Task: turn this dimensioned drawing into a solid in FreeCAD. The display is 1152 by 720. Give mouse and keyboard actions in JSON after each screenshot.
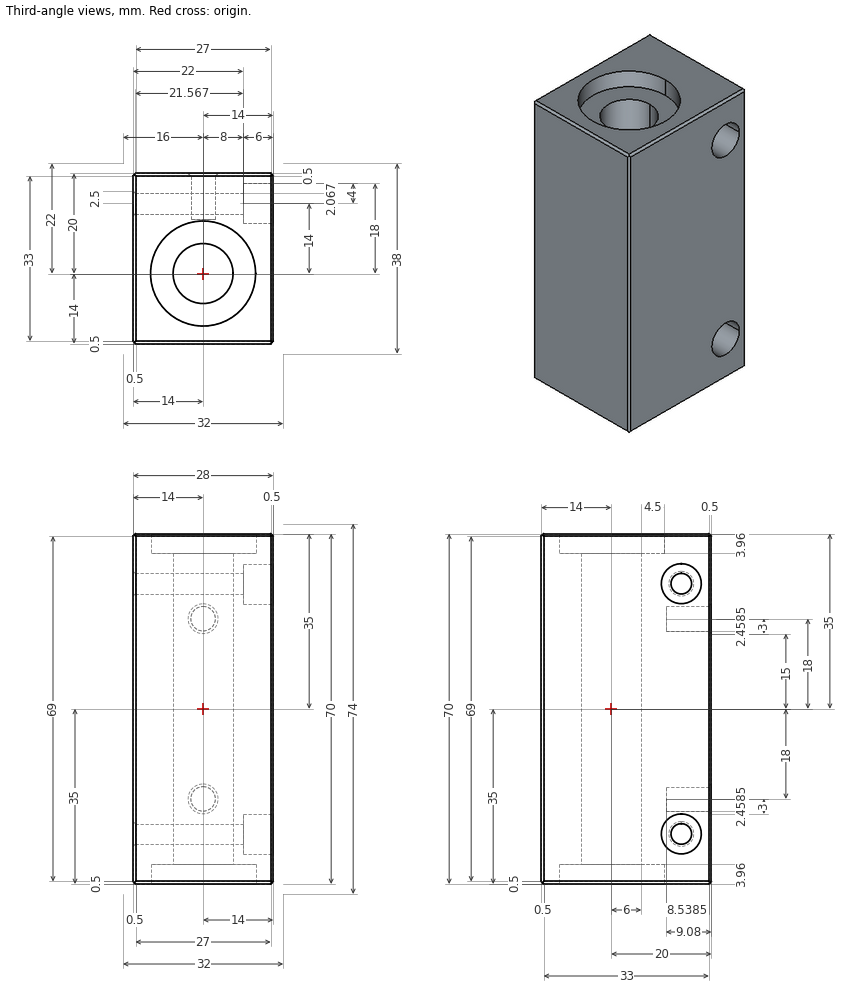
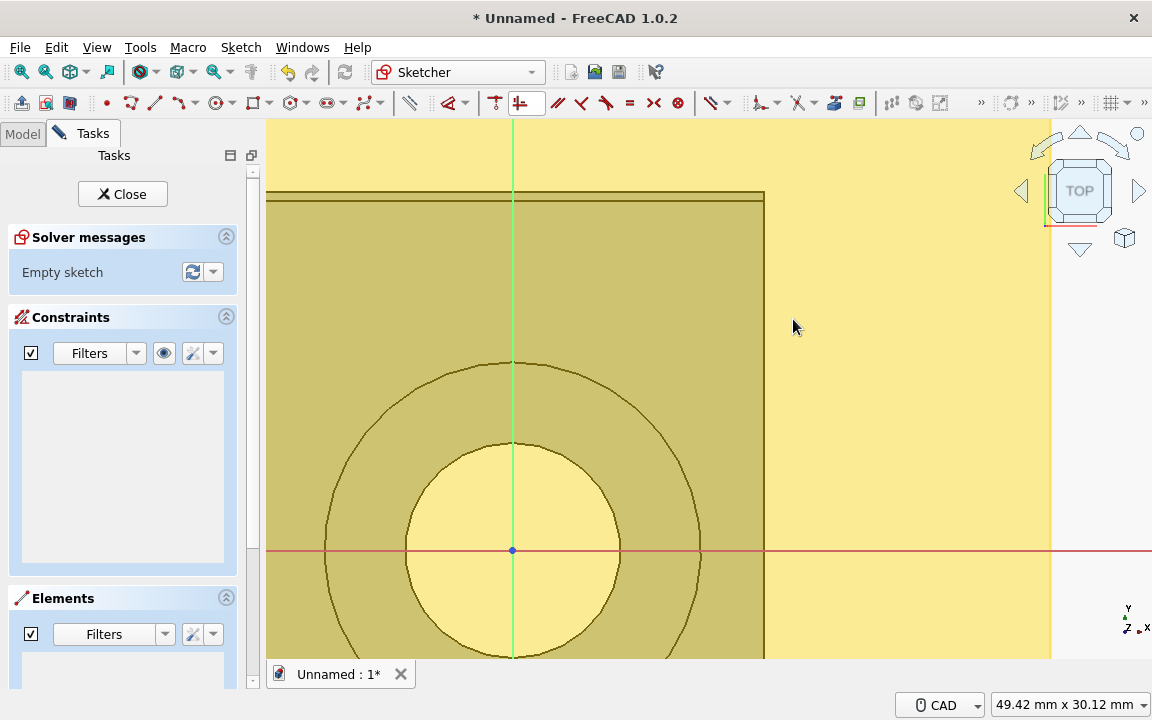
{"action": "key", "text": "g r"}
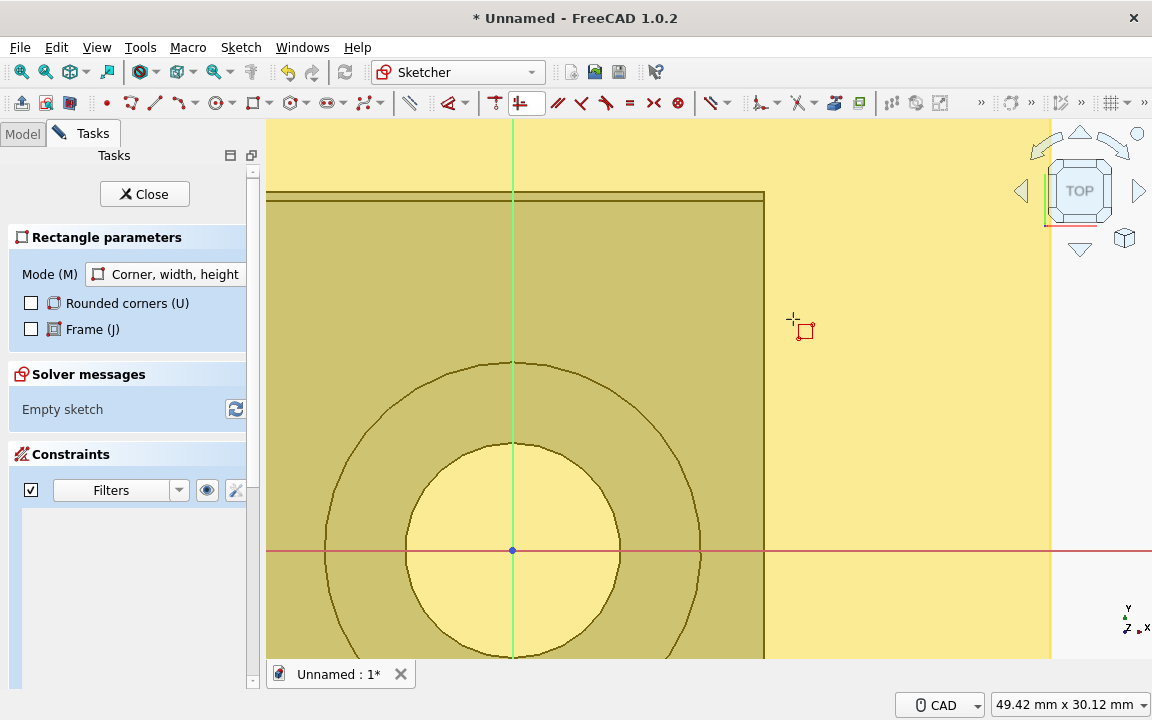
{"action": "left_click", "coordinate": [656, 228]}
{"action": "mouse_move", "coordinate": [764, 300]}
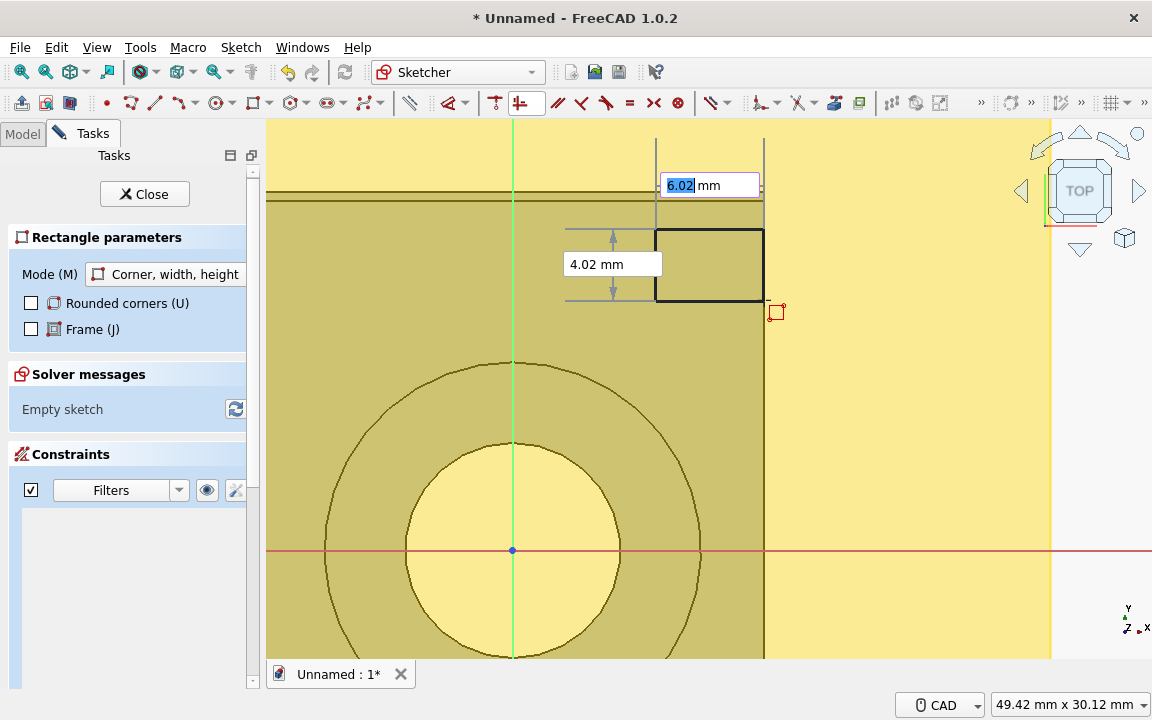
{"action": "type", "text": "6"}
{"action": "key", "text": "Tab"}
{"action": "type", "text": "4"}
{"action": "key", "text": "Return"}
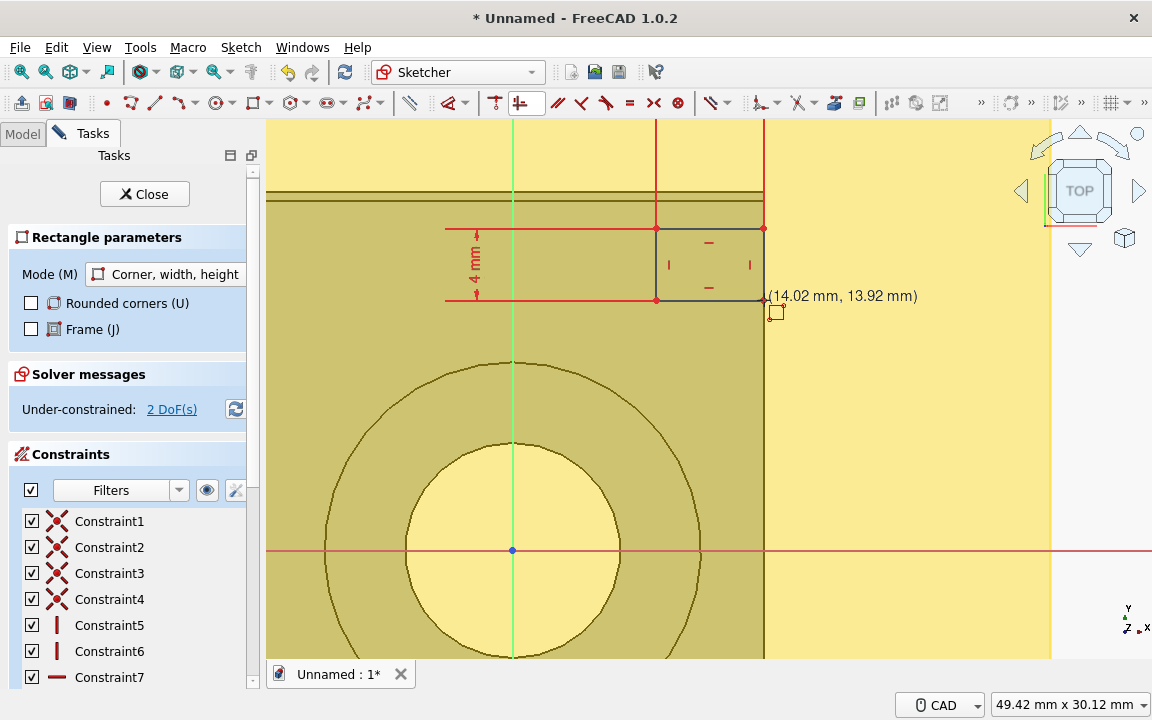
{"action": "left_click", "coordinate": [156, 104]}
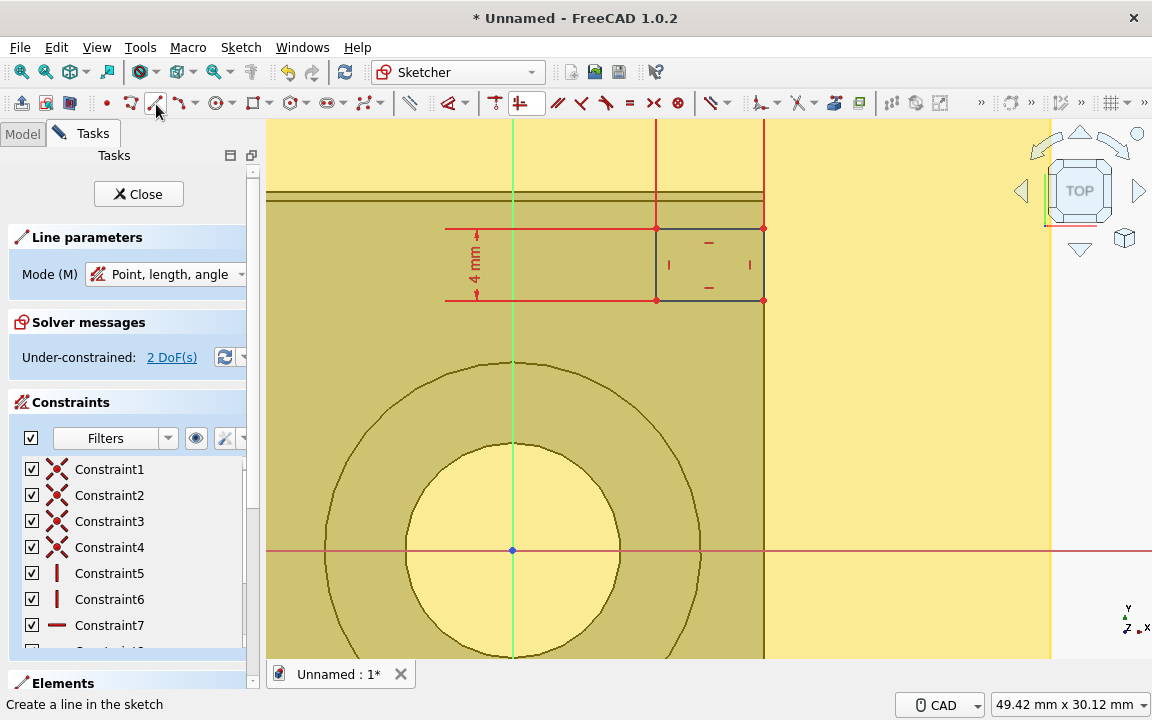
{"action": "scroll", "coordinate": [645, 300], "scroll_direction": "up", "scroll_amount": 2}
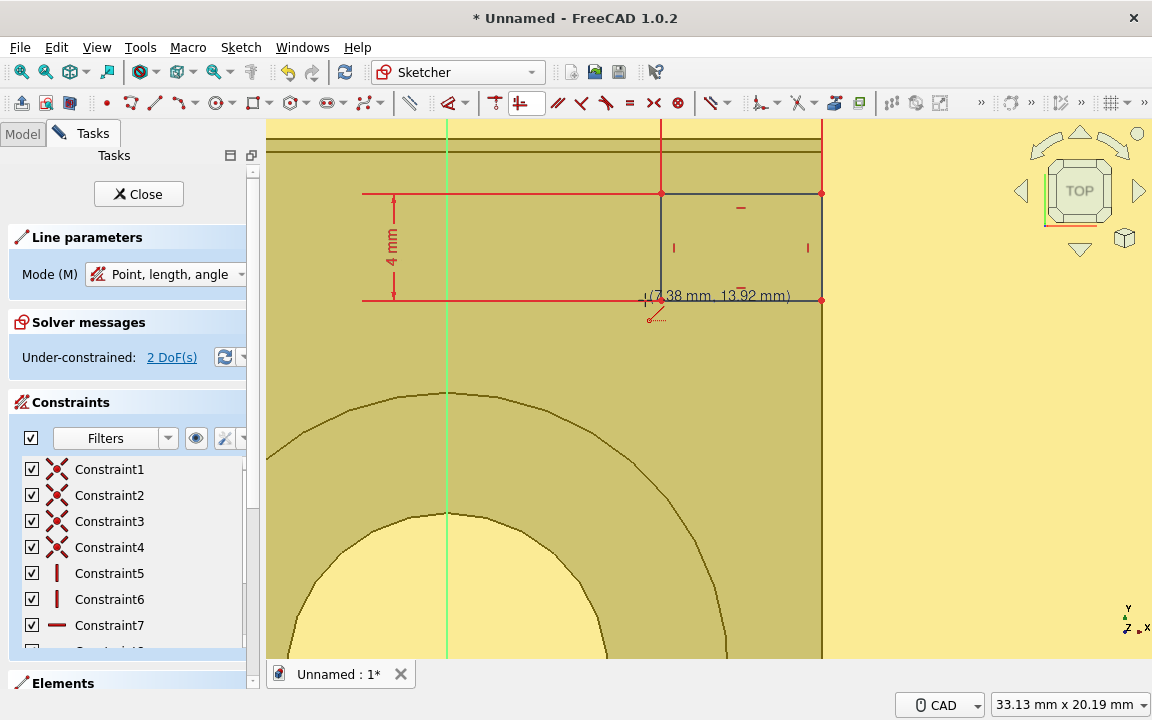
{"action": "left_click", "coordinate": [645, 299]}
{"action": "left_click", "coordinate": [597, 299]}
{"action": "key", "text": "Escape"}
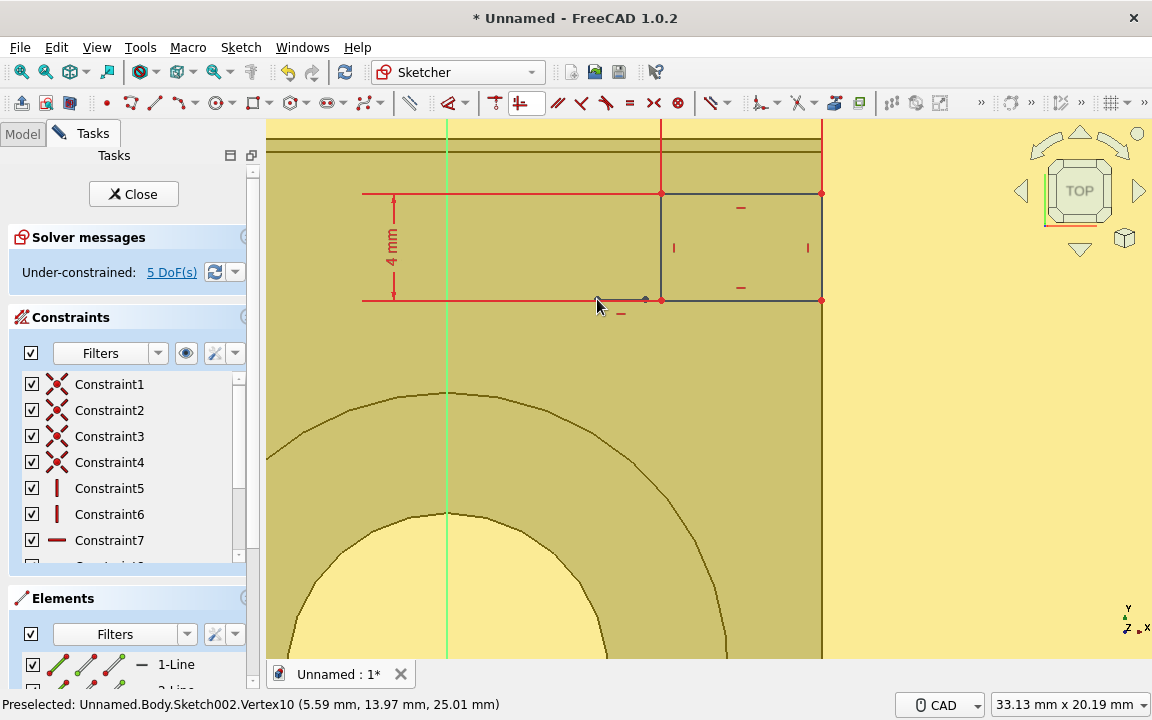
{"action": "left_click", "coordinate": [631, 300]}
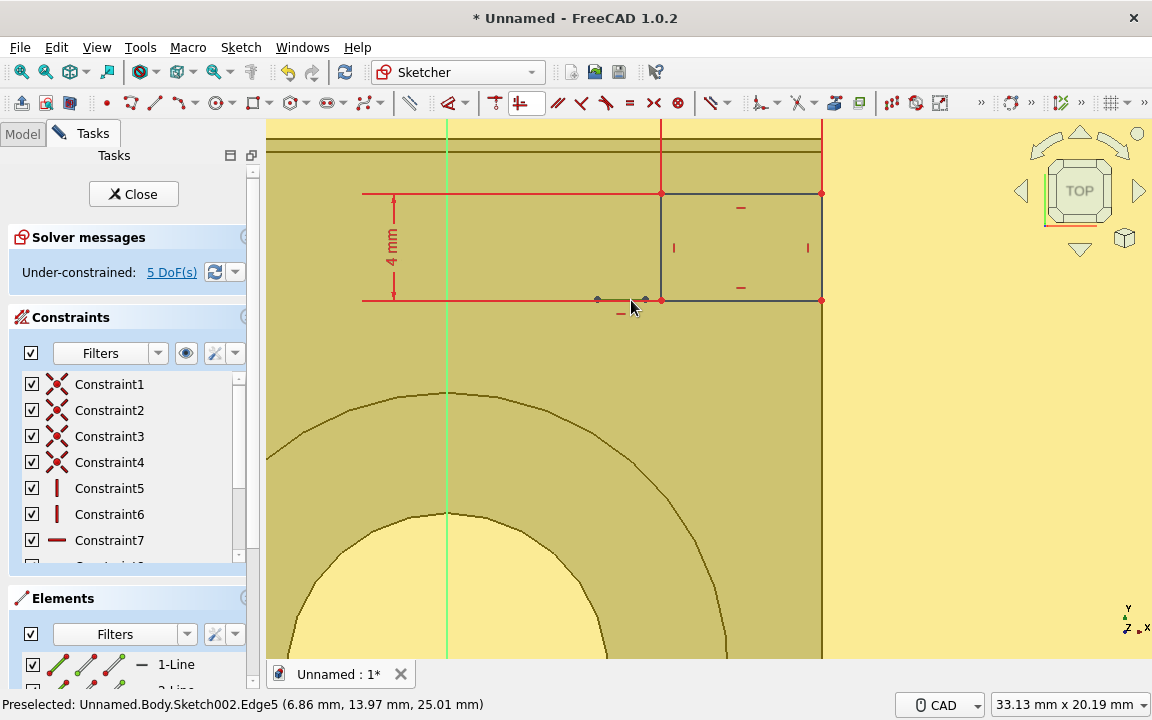
{"action": "left_click", "coordinate": [410, 104]}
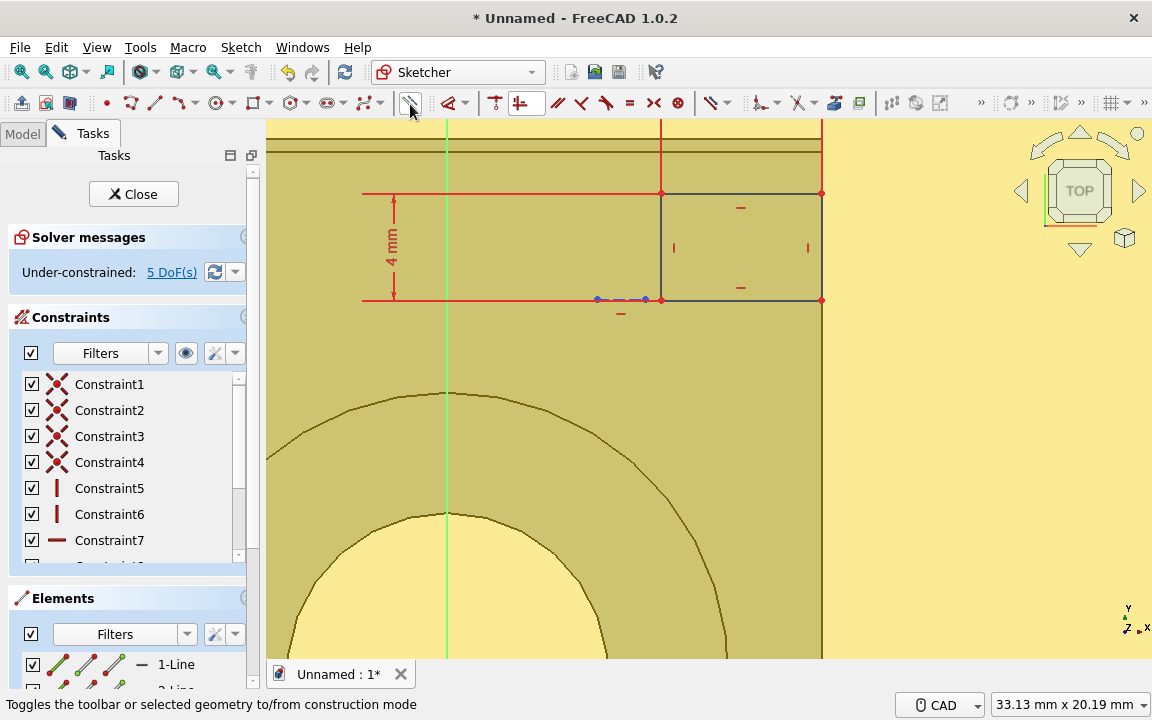
{"action": "left_click", "coordinate": [448, 104]}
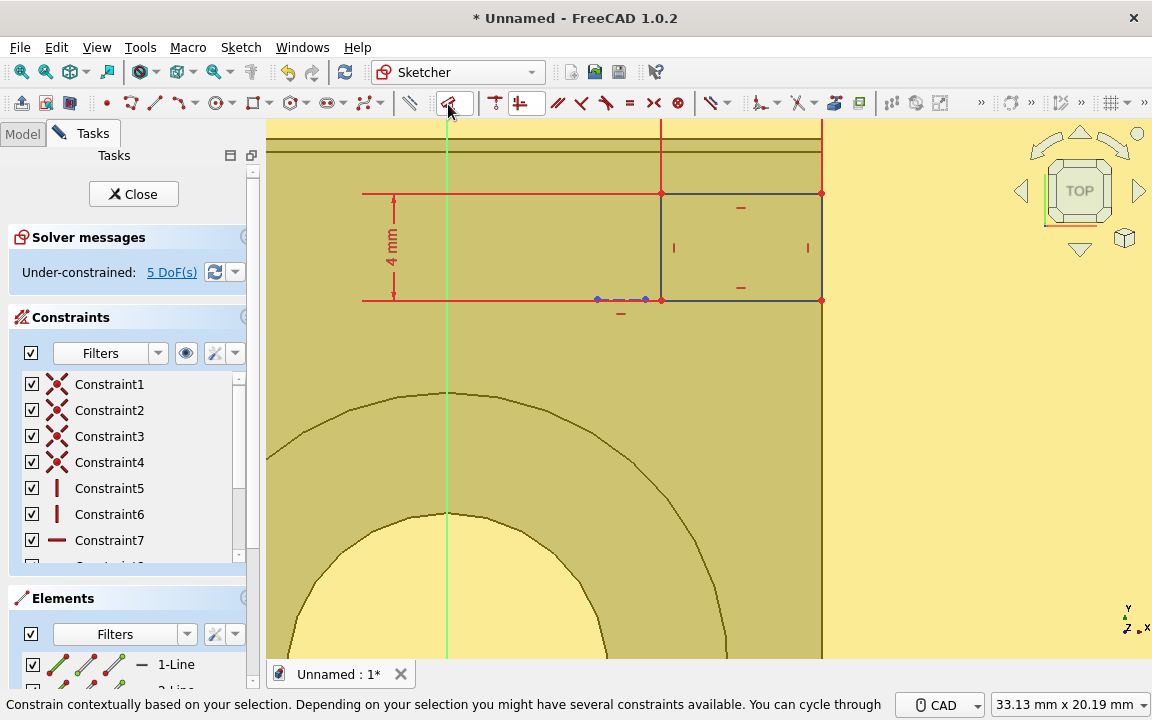
{"action": "left_click", "coordinate": [661, 194]}
{"action": "left_click", "coordinate": [554, 160]}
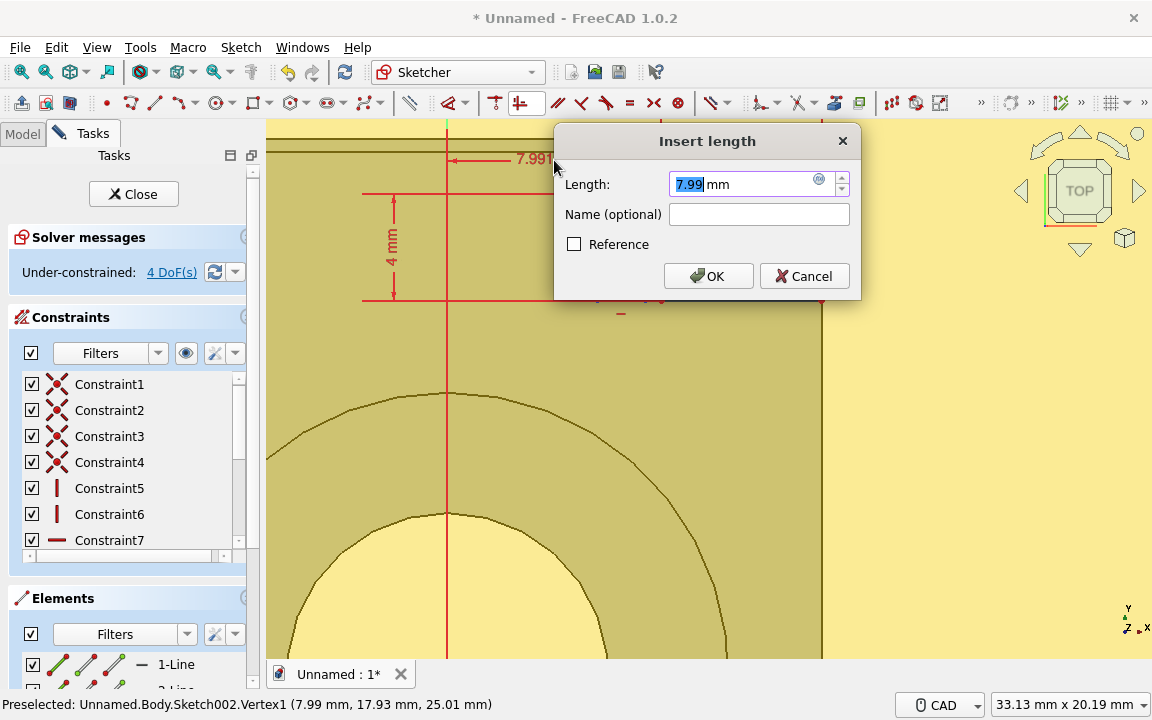
{"action": "type", "text": "8"}
{"action": "key", "text": "Return"}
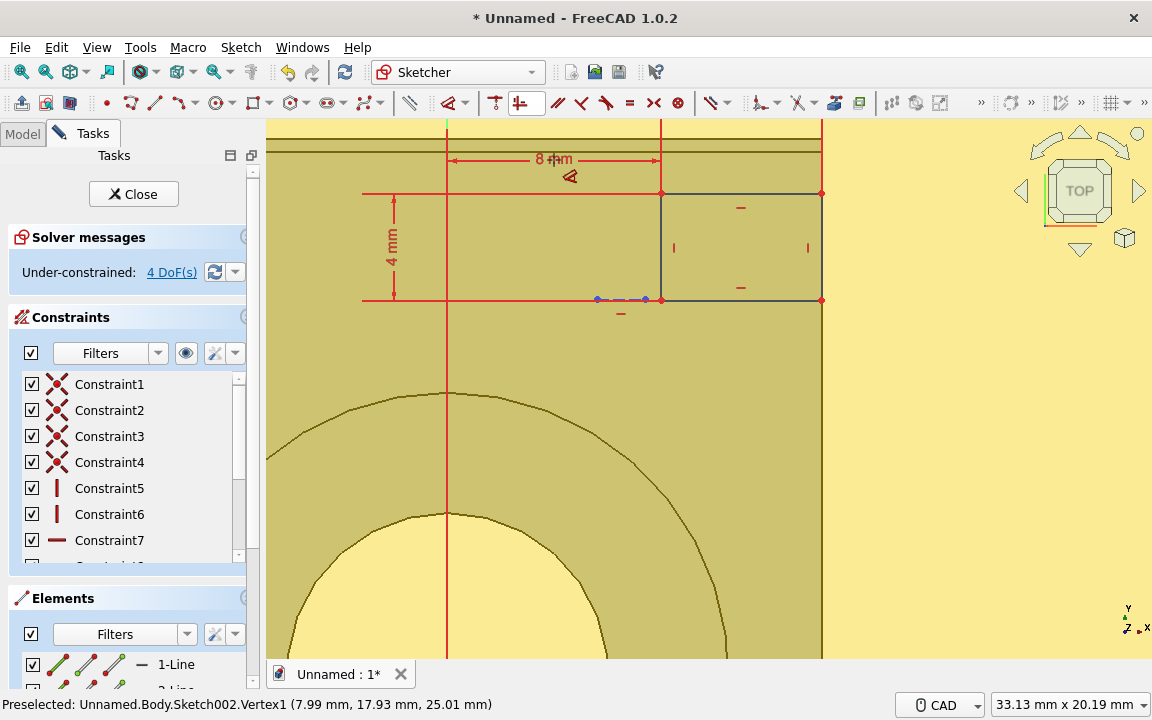
{"action": "left_click", "coordinate": [661, 194]}
{"action": "left_click", "coordinate": [413, 412]}